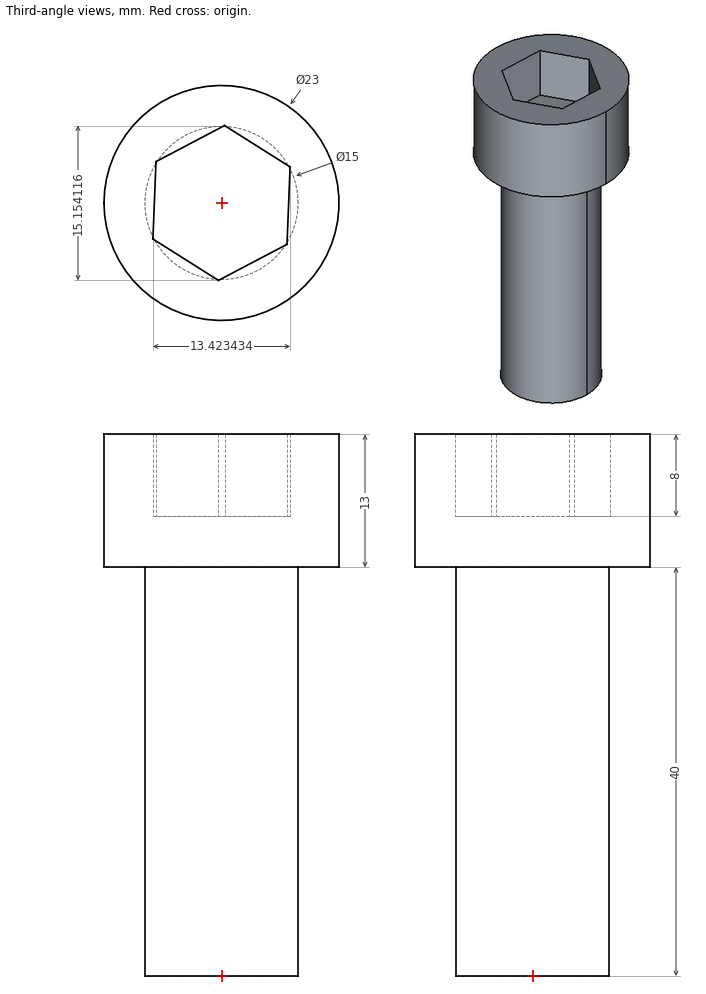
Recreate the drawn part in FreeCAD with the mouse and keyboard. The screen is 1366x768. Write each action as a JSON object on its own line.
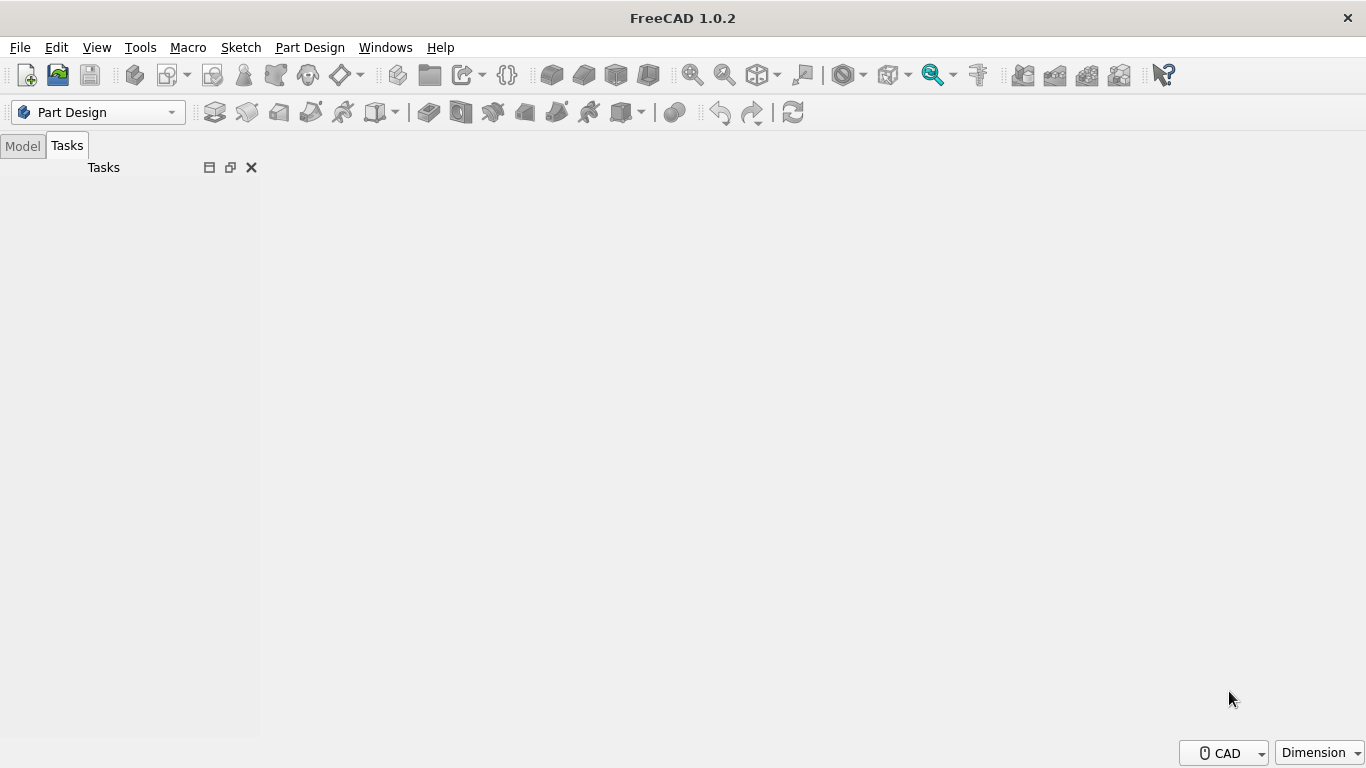
{"action": "left_click", "coordinate": [26, 76]}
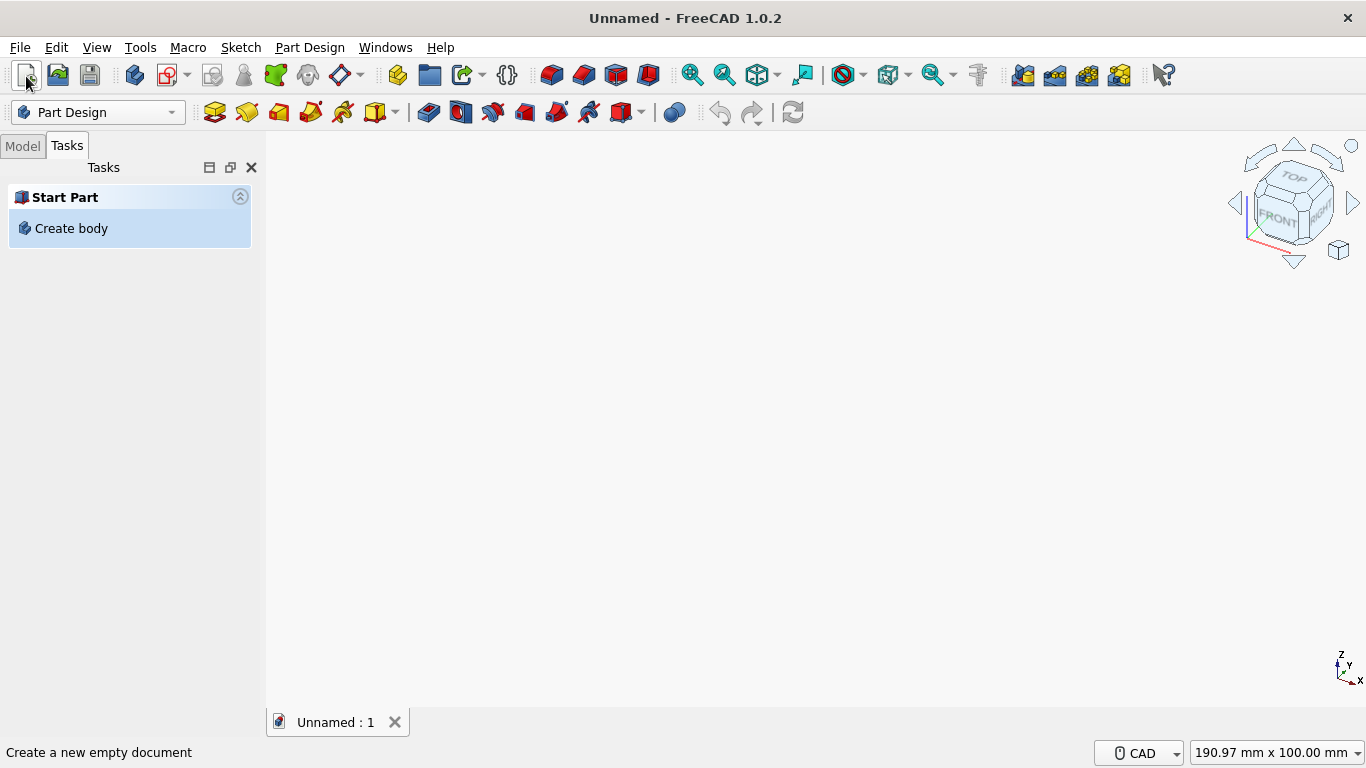
{"action": "left_click", "coordinate": [168, 76]}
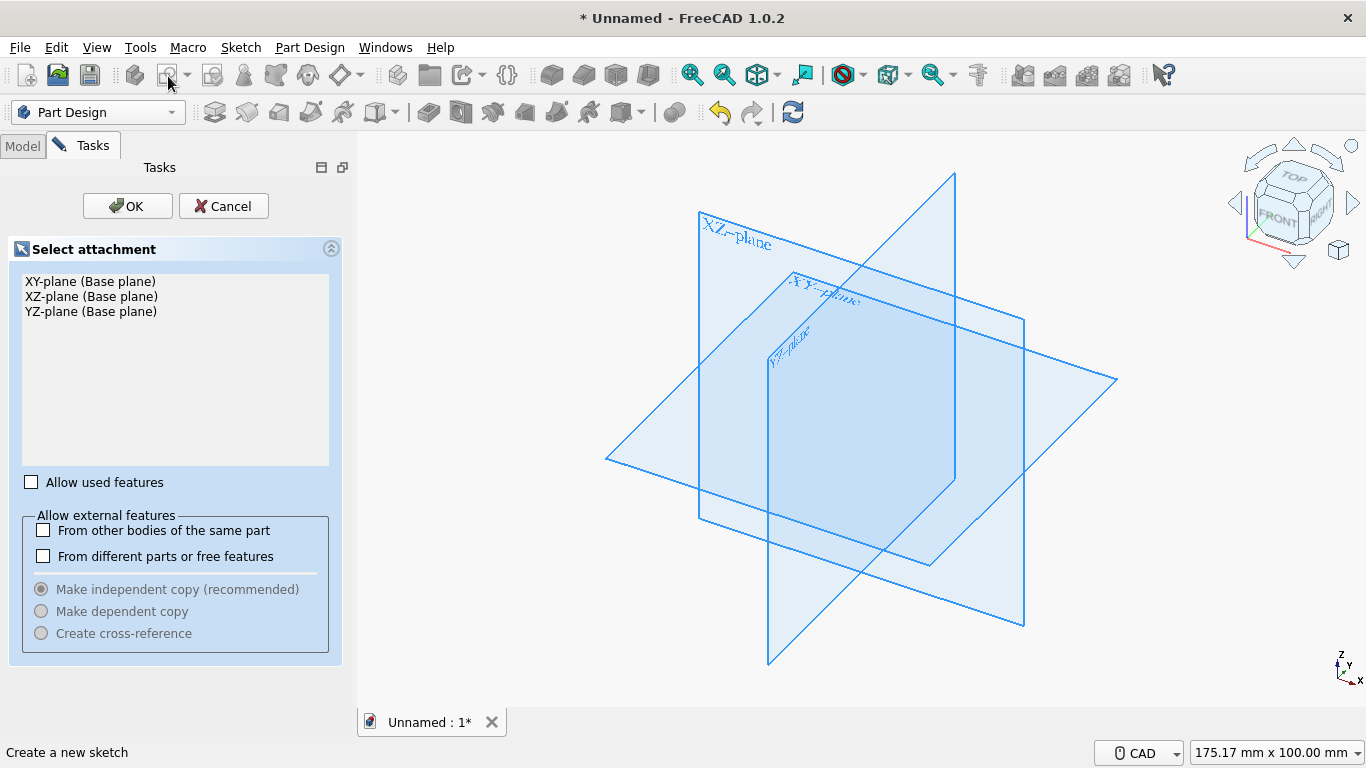
{"action": "left_click", "coordinate": [82, 282]}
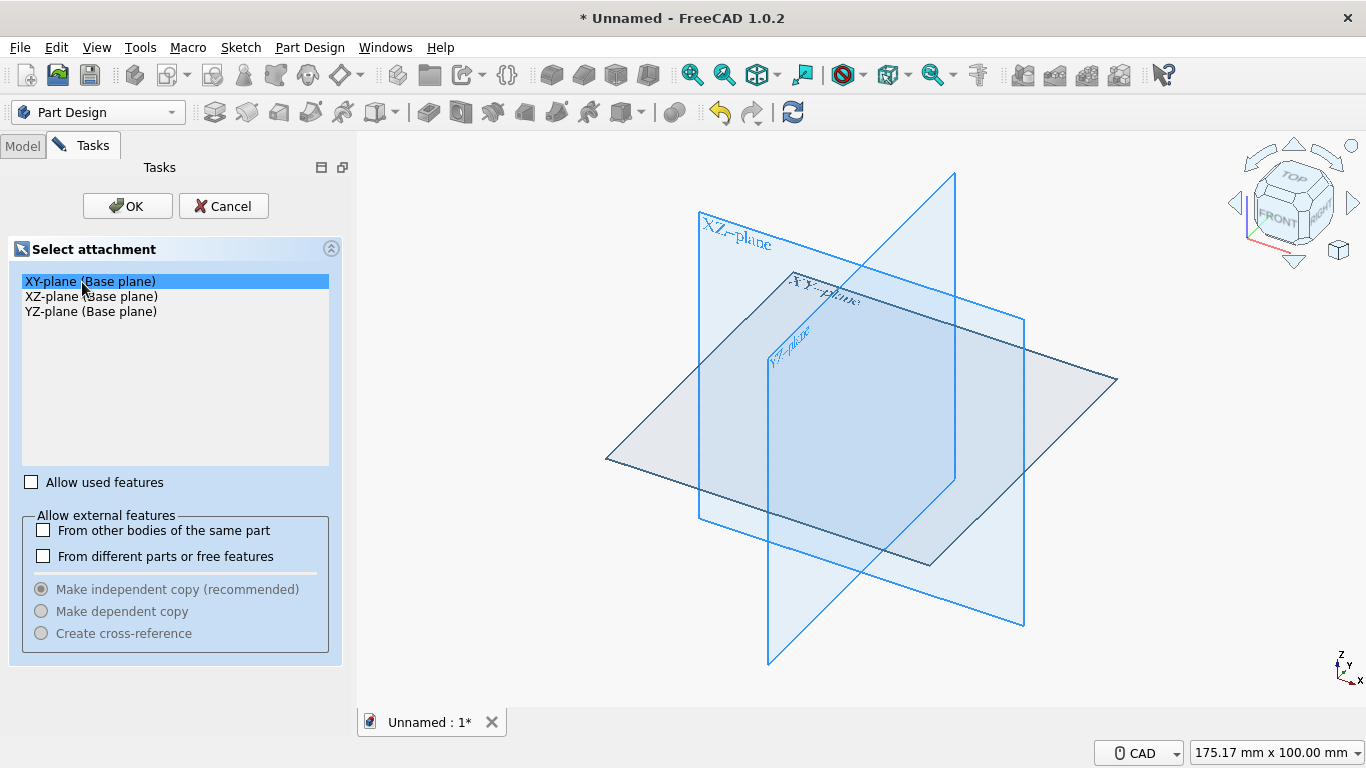
{"action": "left_click", "coordinate": [128, 206]}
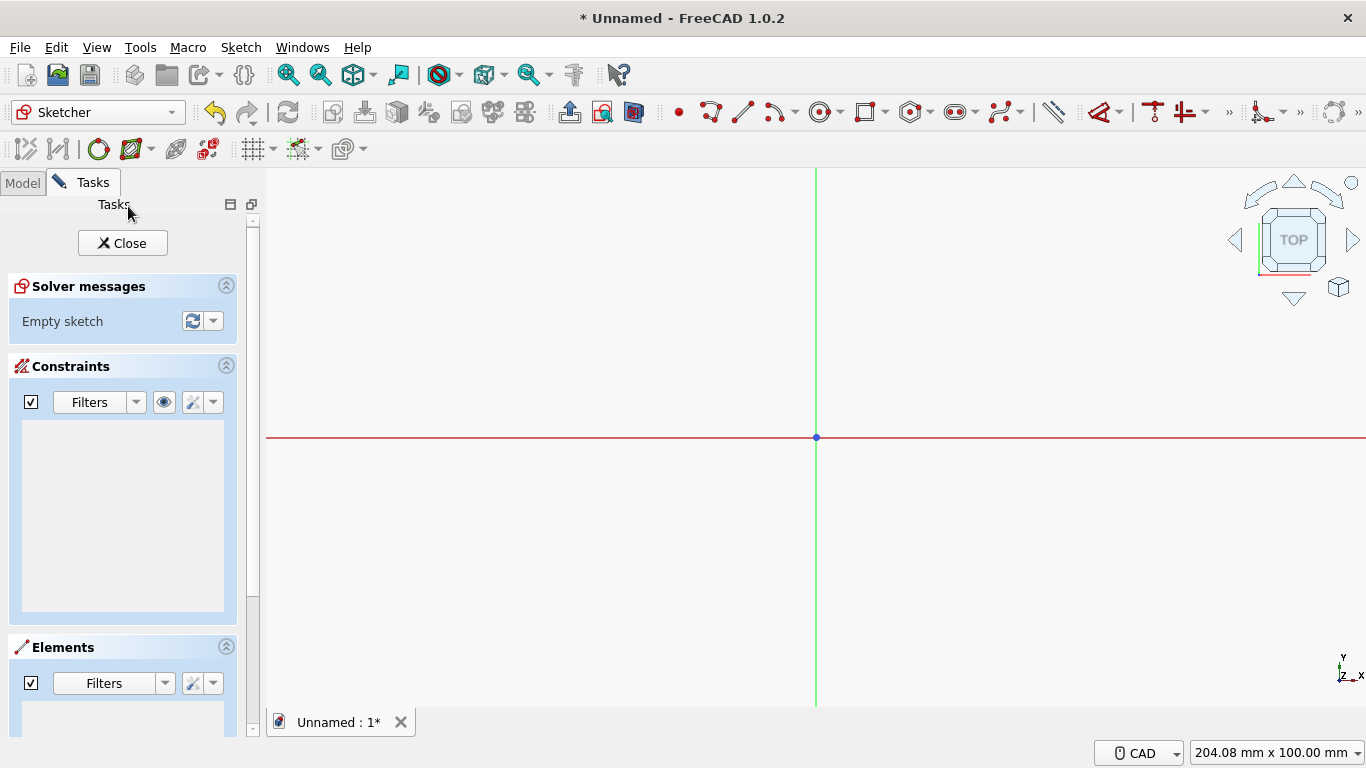
{"action": "scroll", "coordinate": [838, 438], "scroll_direction": "up", "scroll_amount": 7}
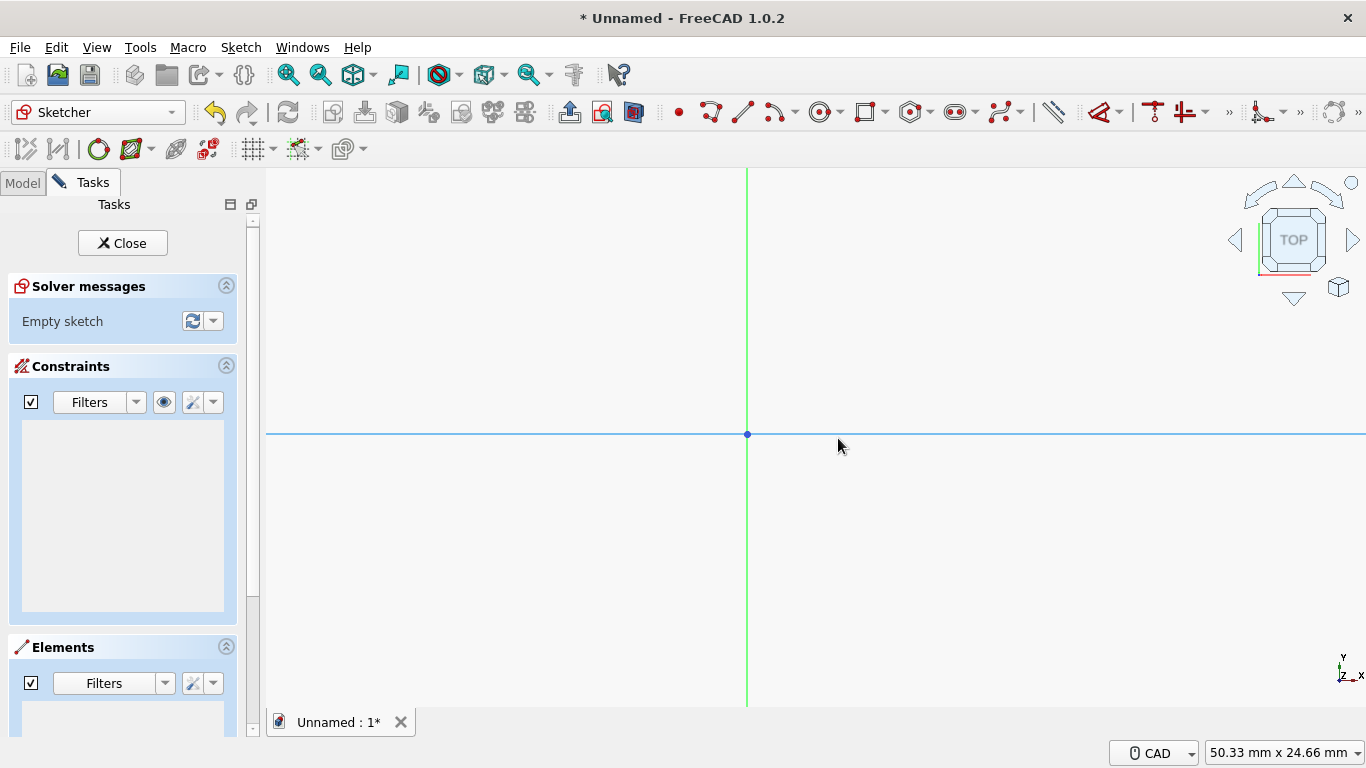
{"action": "left_click", "coordinate": [820, 112]}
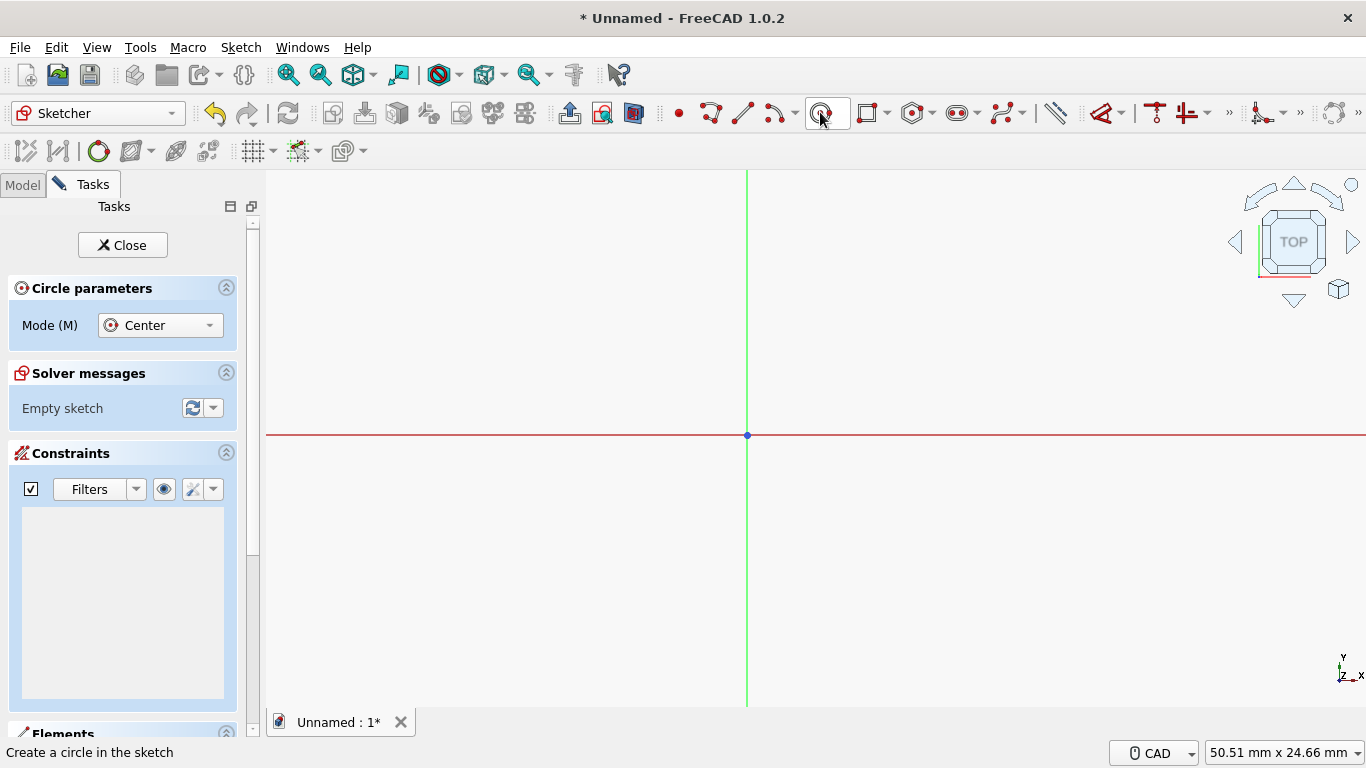
{"action": "left_click", "coordinate": [747, 435]}
{"action": "left_click", "coordinate": [863, 320]}
{"action": "key", "text": "Escape"}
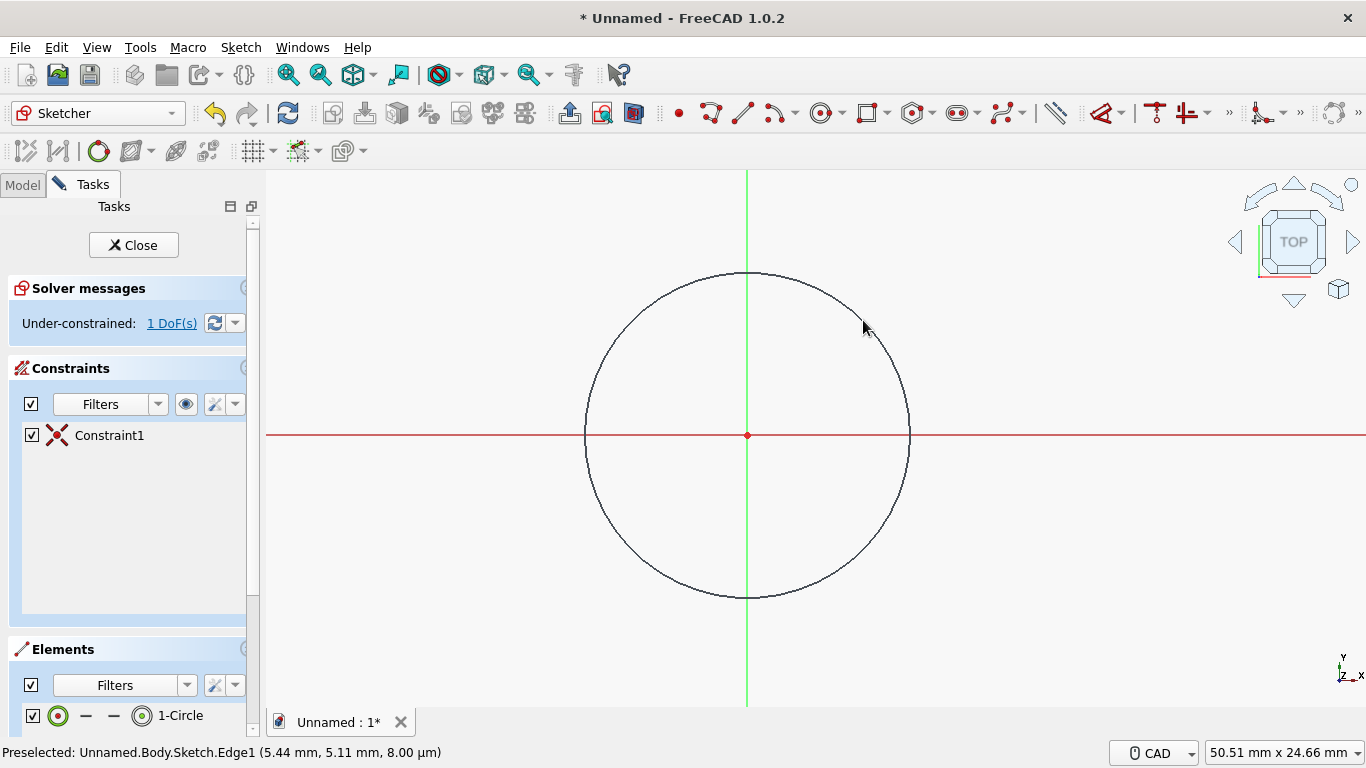
{"action": "left_click", "coordinate": [1102, 114]}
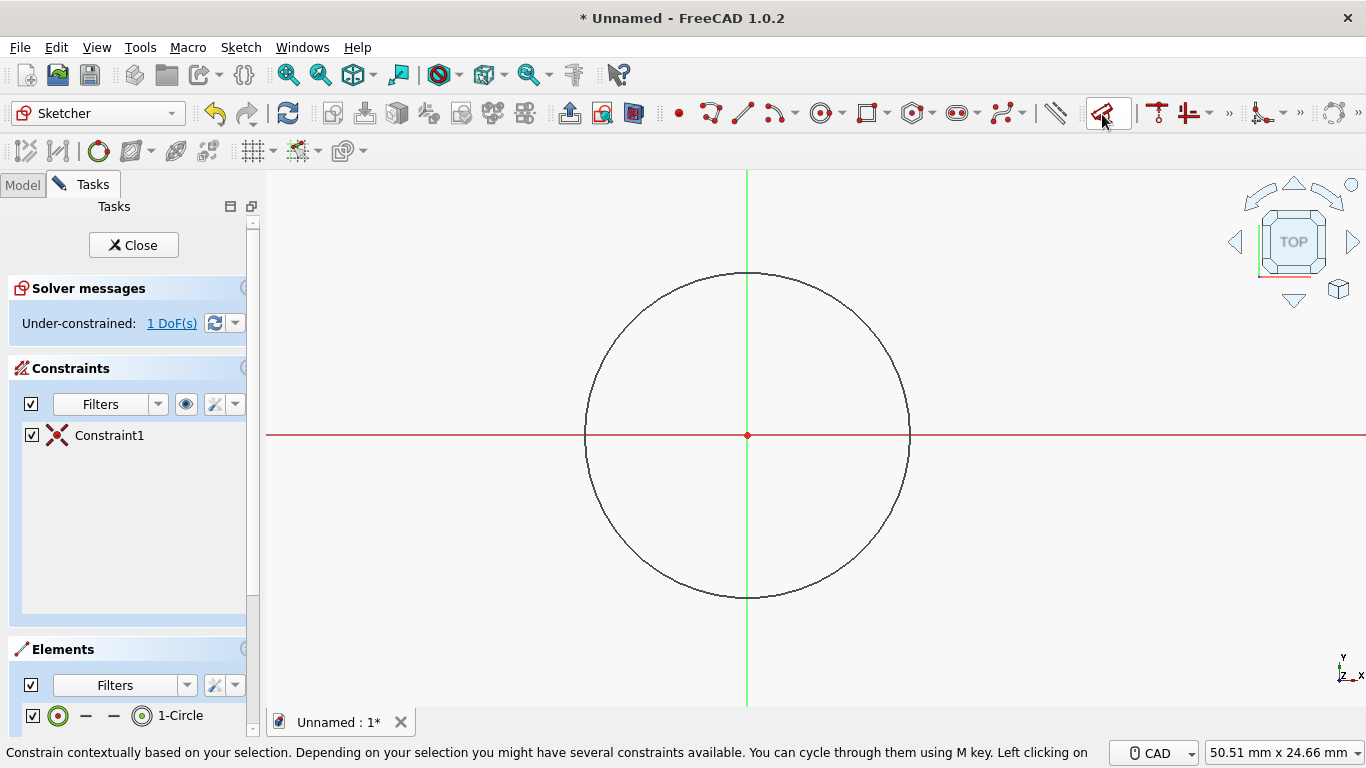
{"action": "left_click", "coordinate": [862, 320]}
{"action": "left_click", "coordinate": [885, 297]}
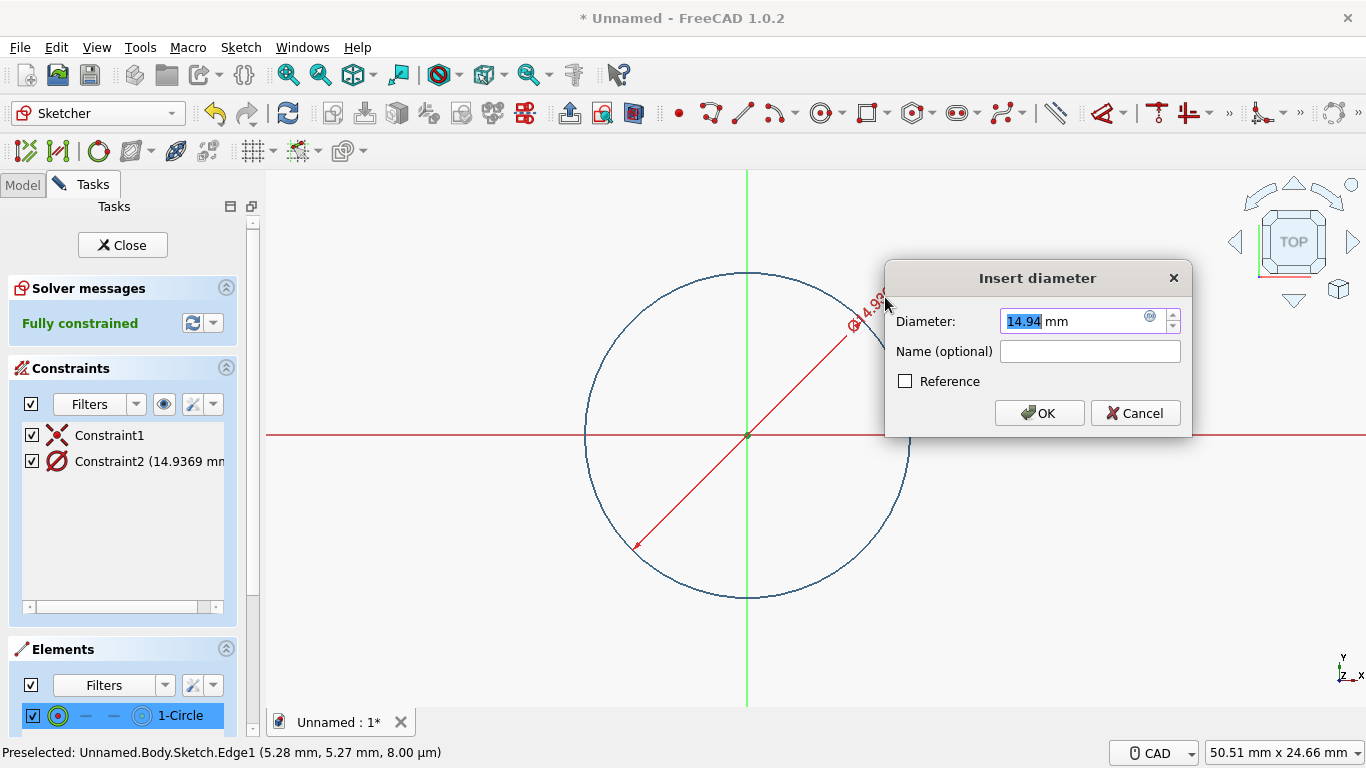
{"action": "type", "text": "15"}
{"action": "key", "text": "Return"}
{"action": "key", "text": "Escape"}